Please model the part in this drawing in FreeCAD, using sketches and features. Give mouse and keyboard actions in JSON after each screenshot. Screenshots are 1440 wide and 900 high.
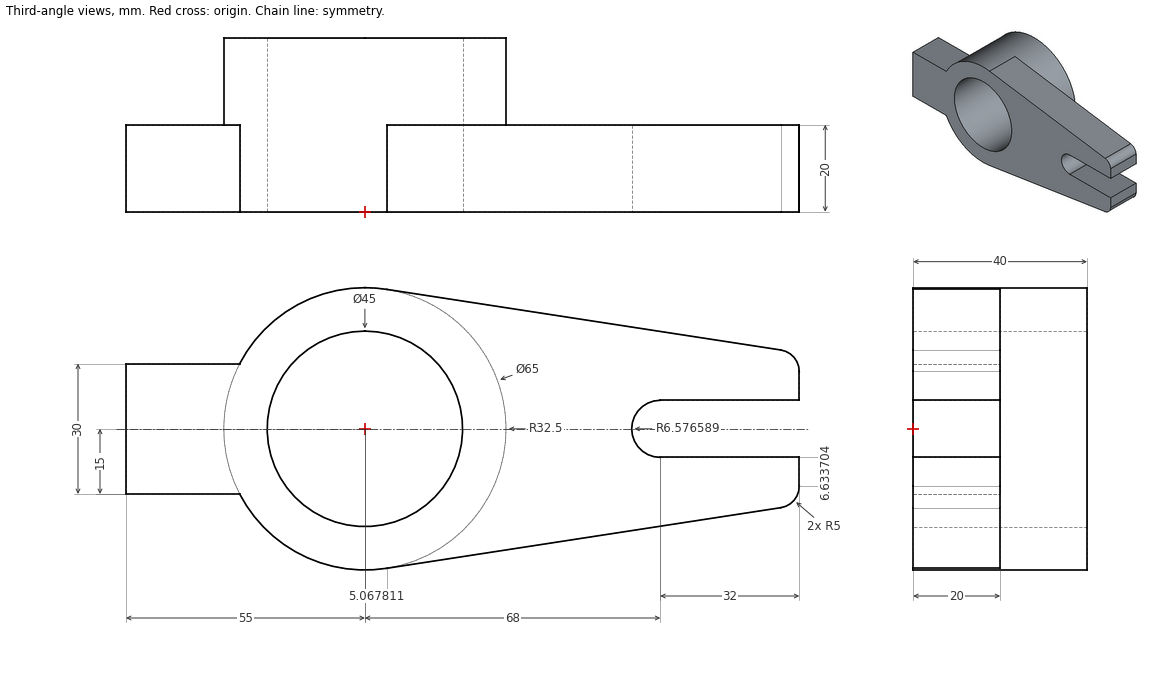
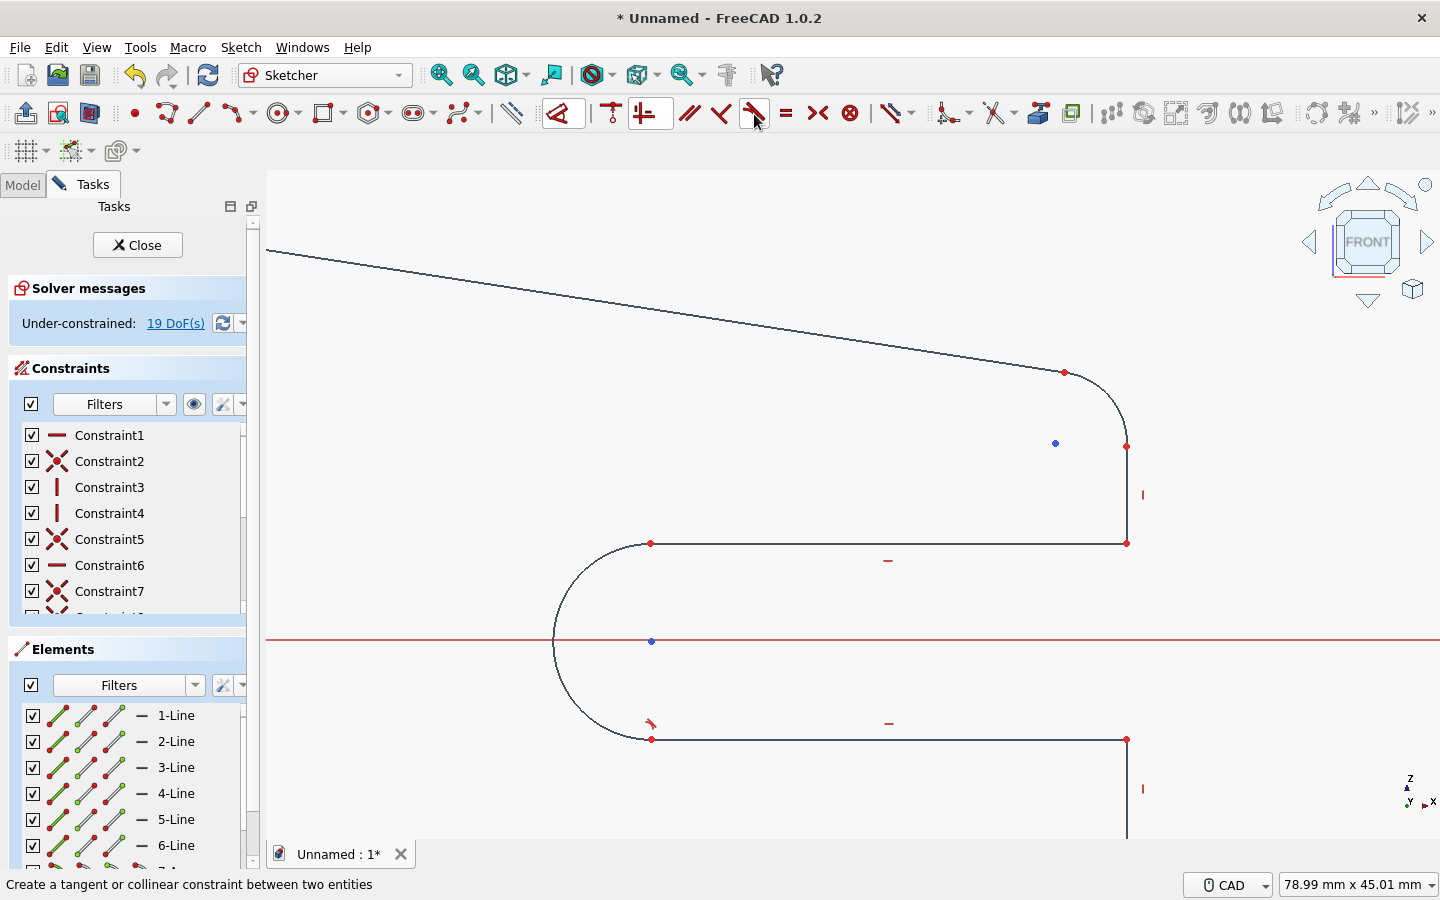
{"action": "left_click", "coordinate": [1127, 769]}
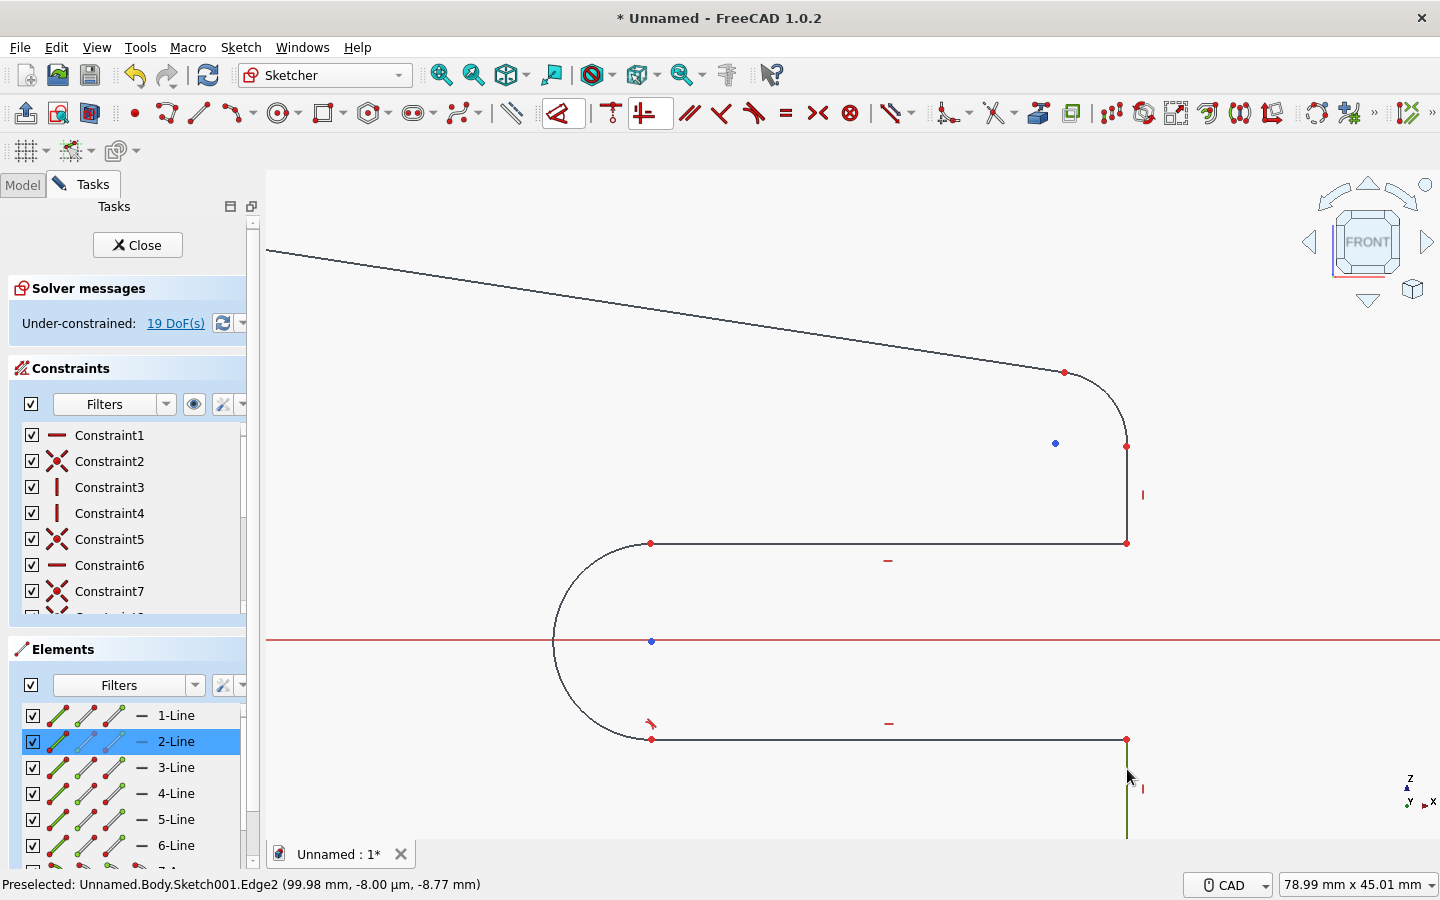
{"action": "scroll", "coordinate": [1111, 394], "scroll_direction": "down", "scroll_amount": 4}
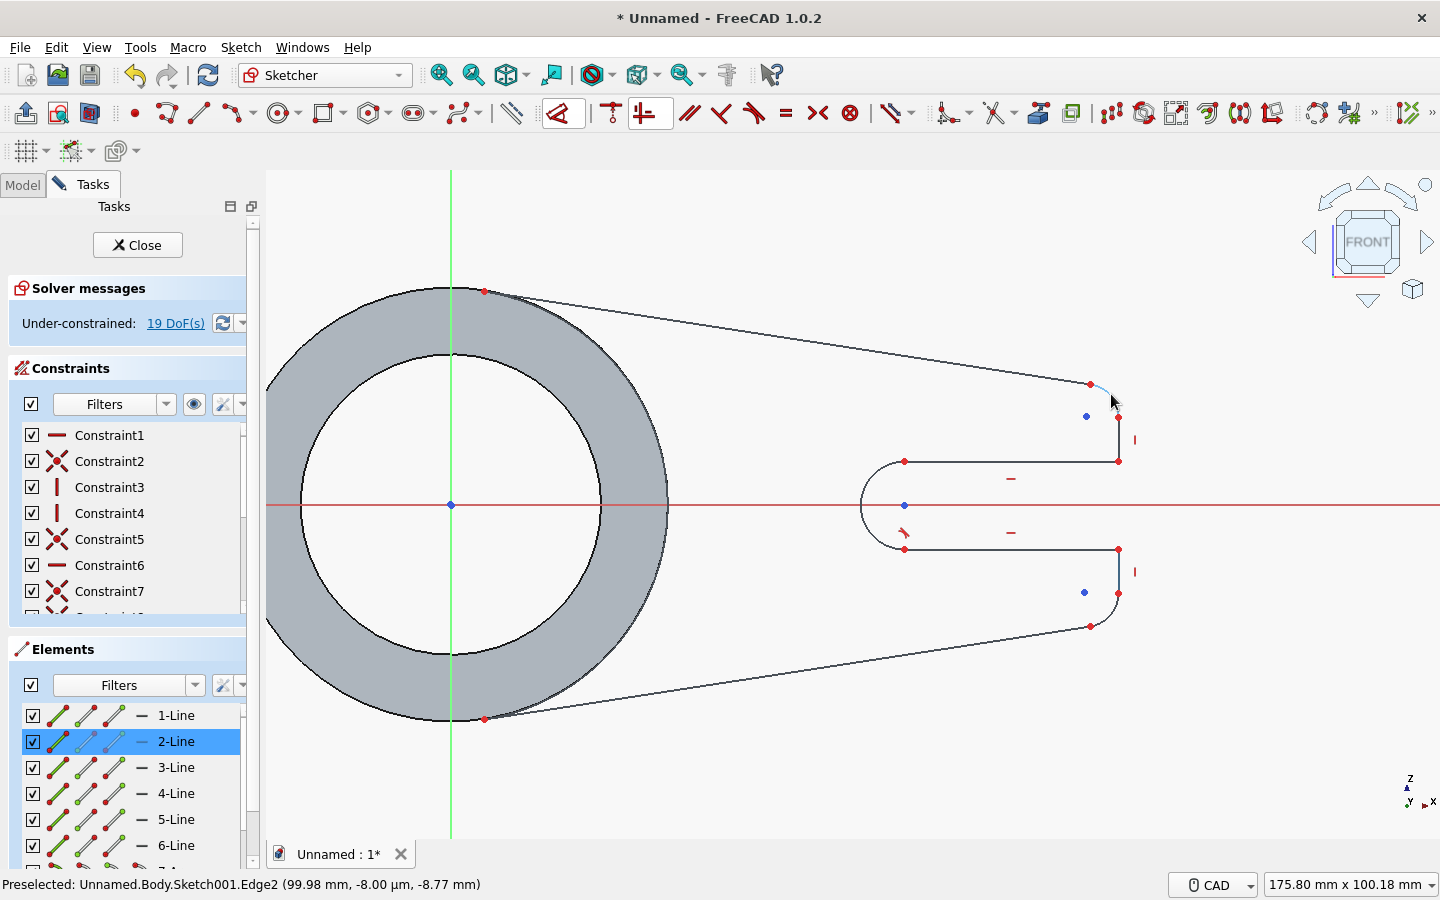
{"action": "left_click", "coordinate": [1103, 621]}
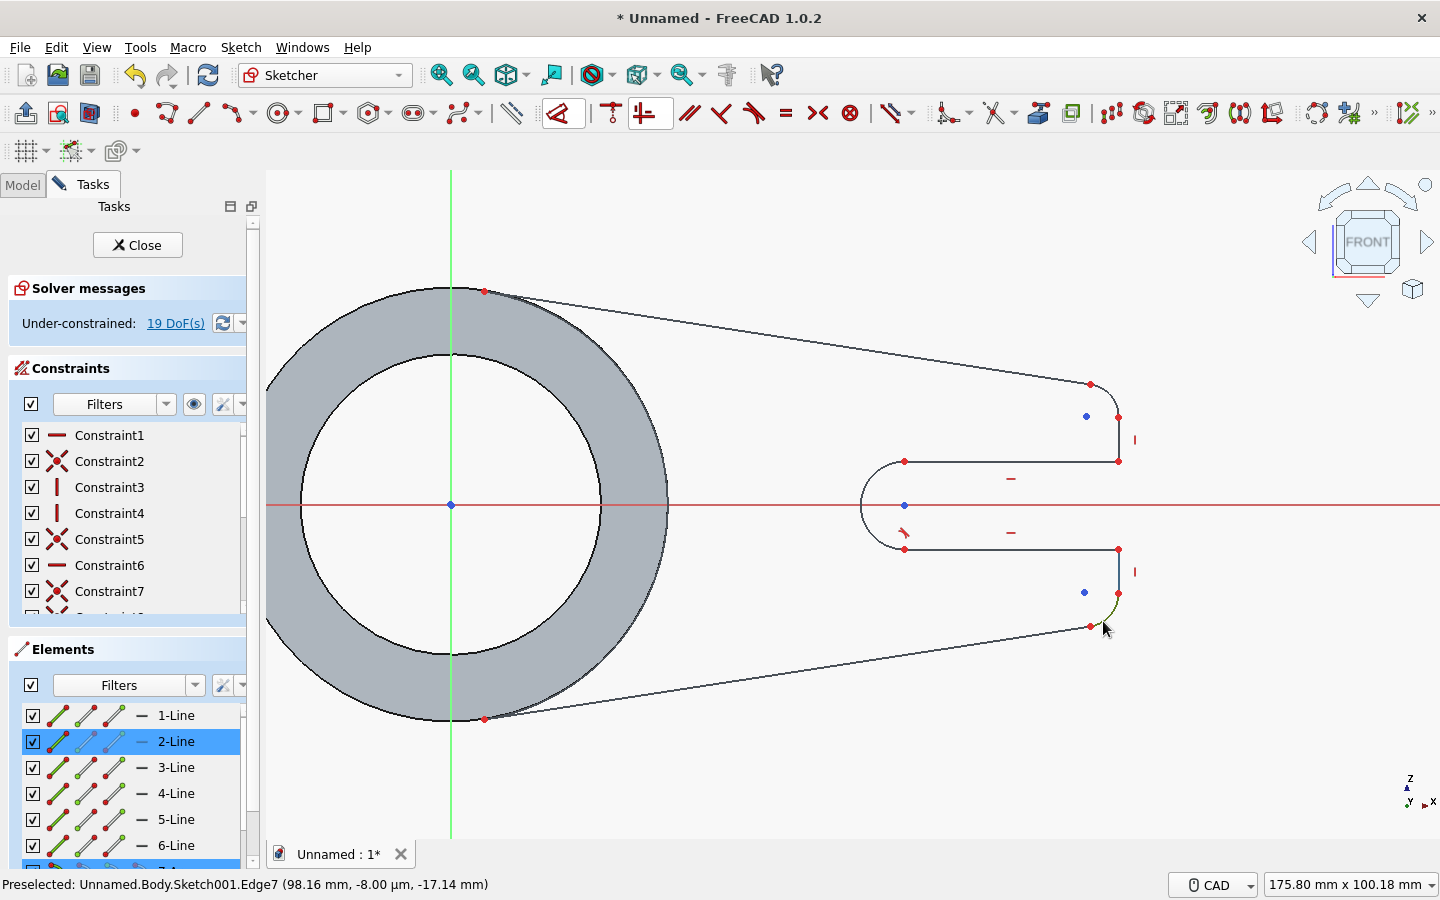
{"action": "left_click", "coordinate": [754, 114]}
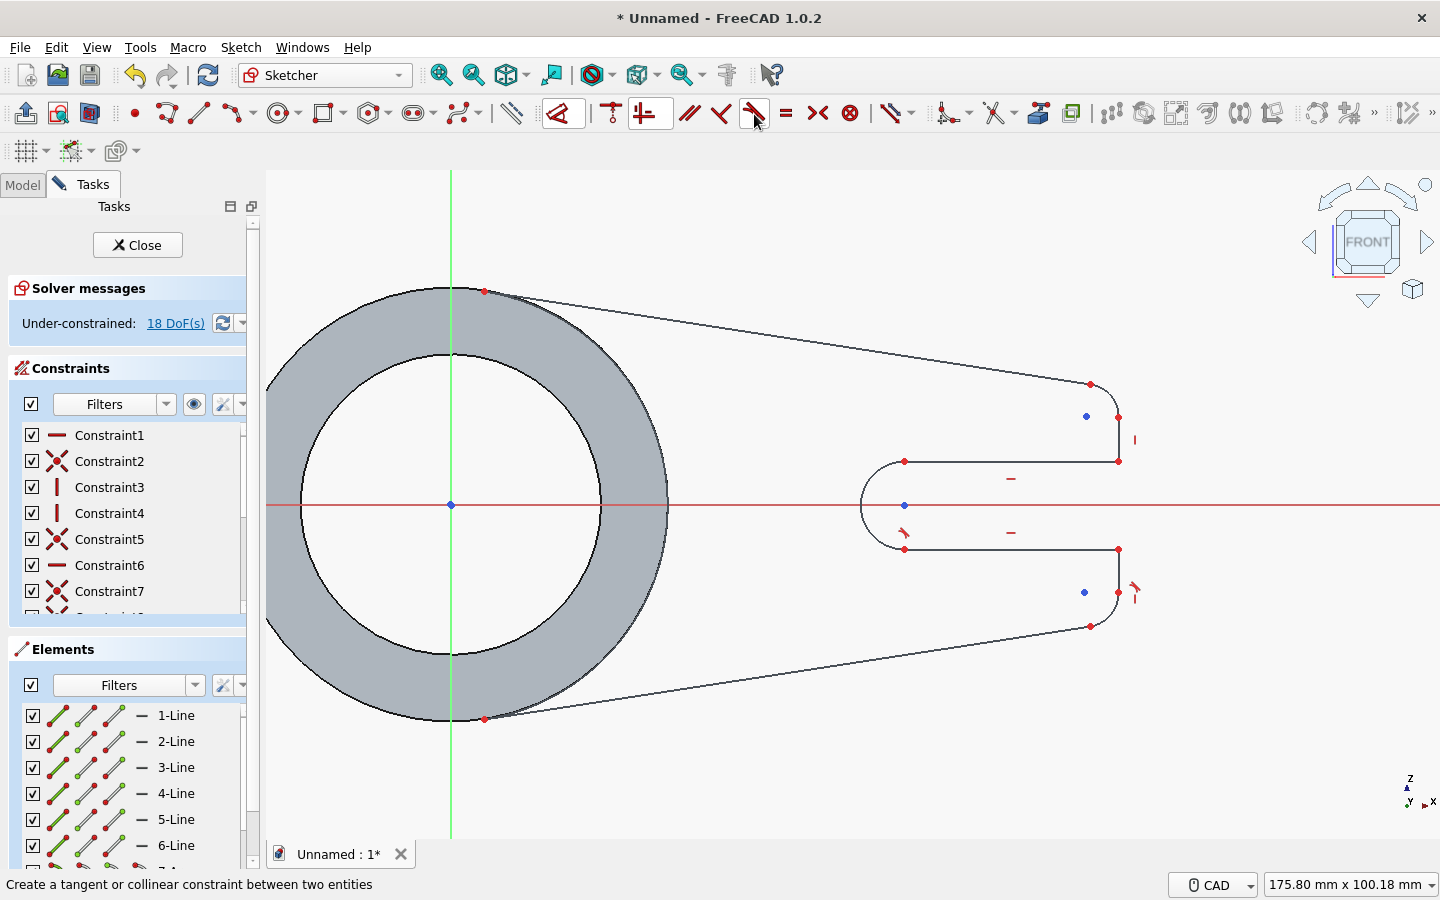
{"action": "left_click", "coordinate": [909, 654]}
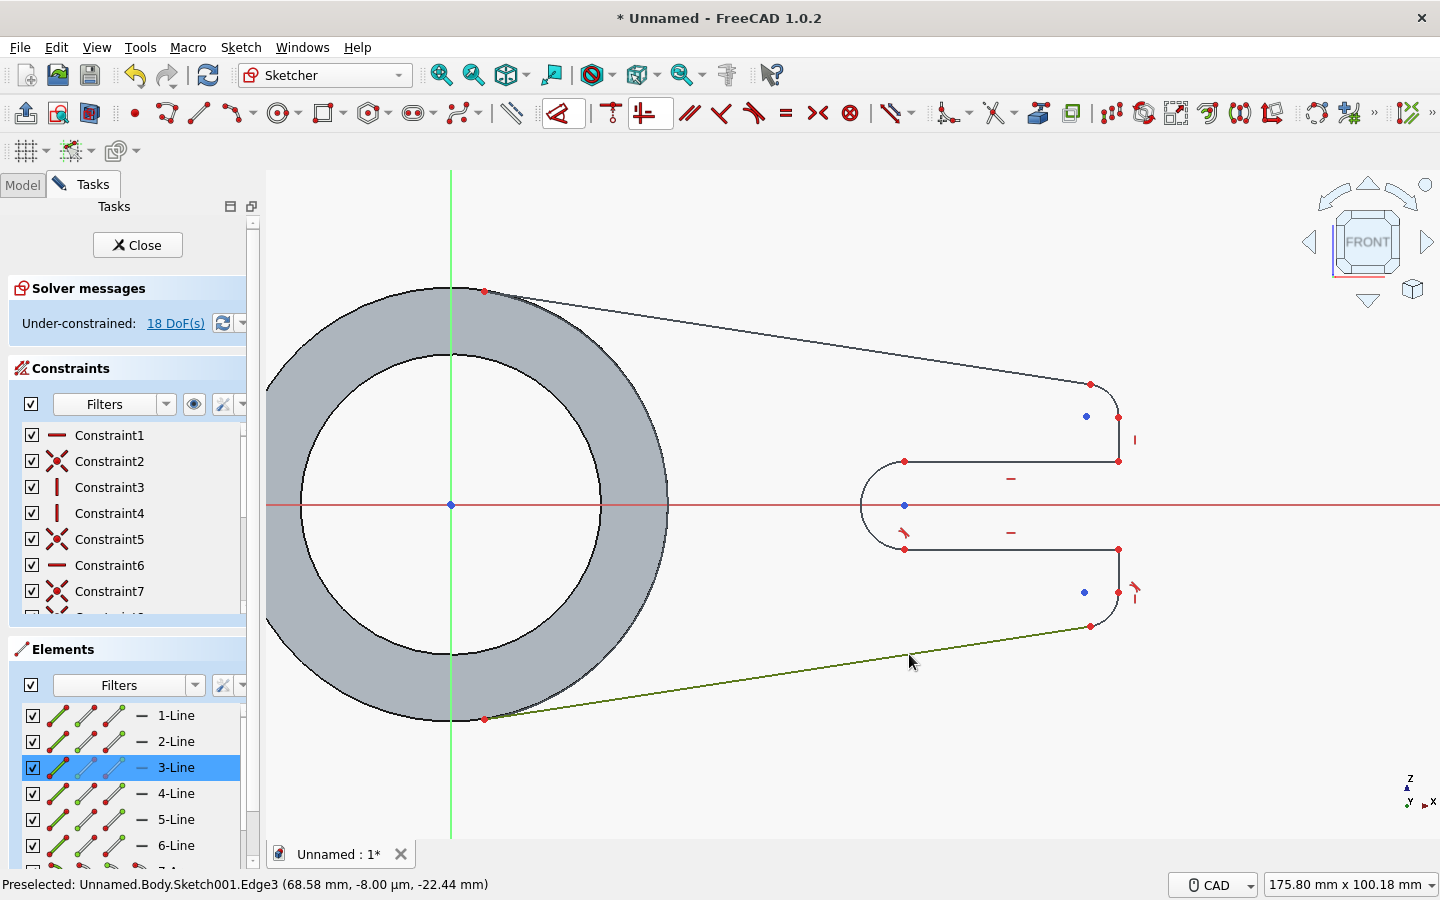
{"action": "left_click", "coordinate": [1104, 621]}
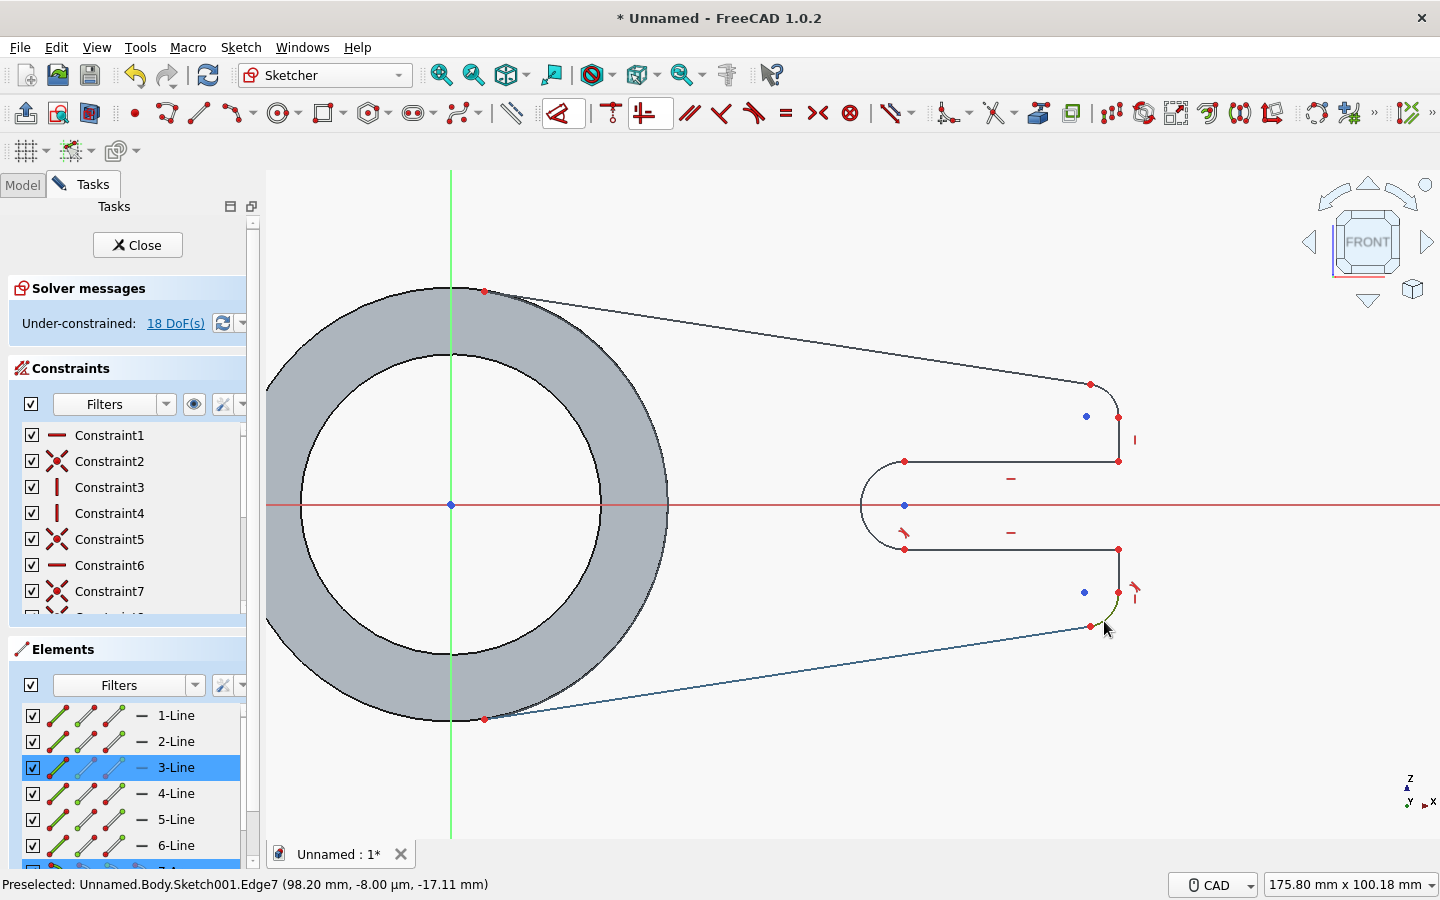
{"action": "left_click", "coordinate": [754, 114]}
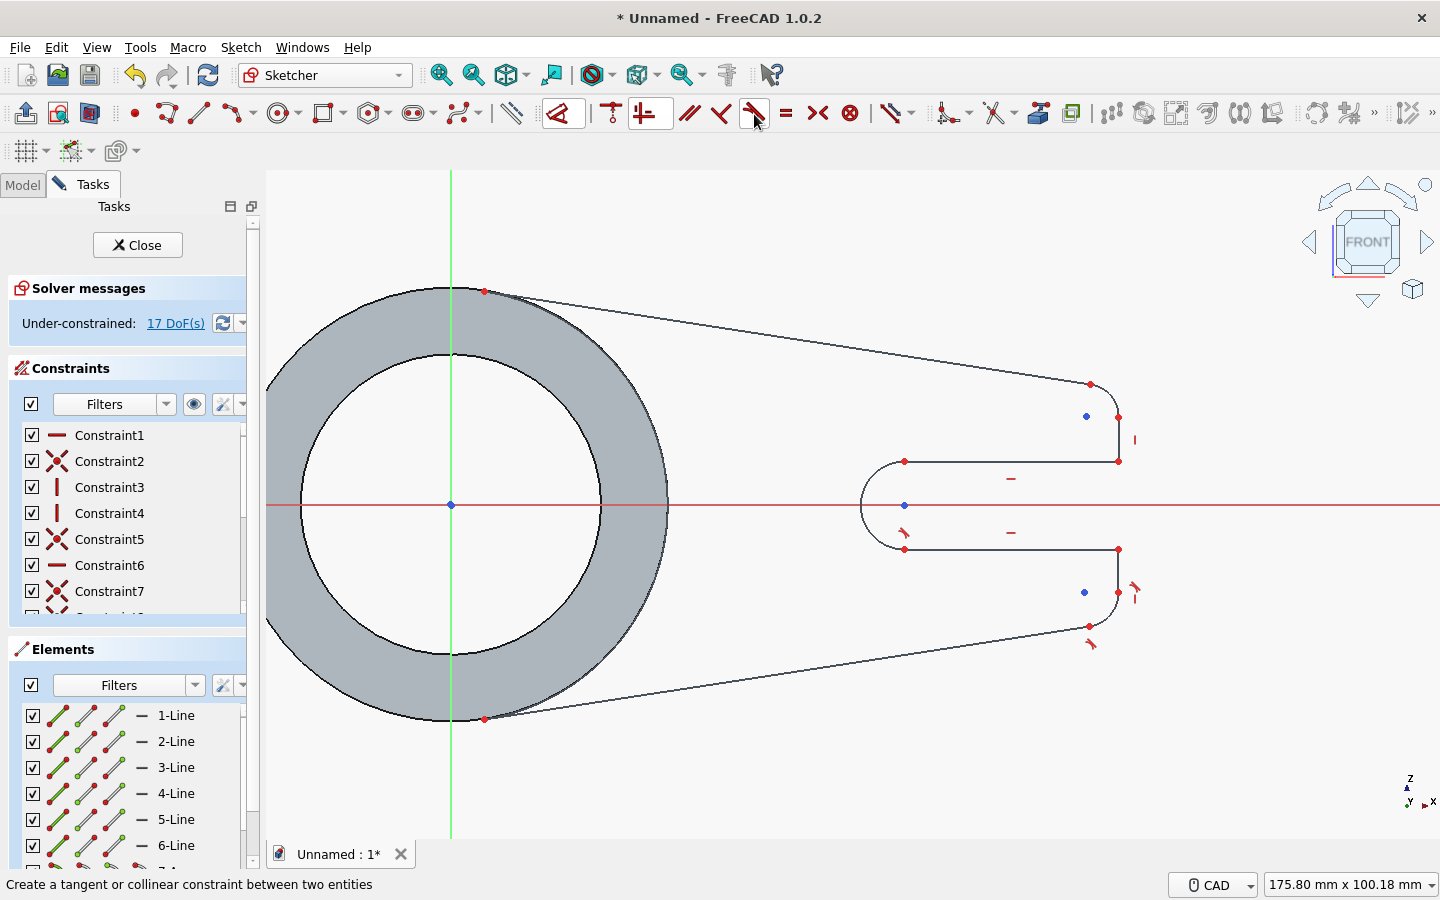
{"action": "left_click", "coordinate": [666, 319]}